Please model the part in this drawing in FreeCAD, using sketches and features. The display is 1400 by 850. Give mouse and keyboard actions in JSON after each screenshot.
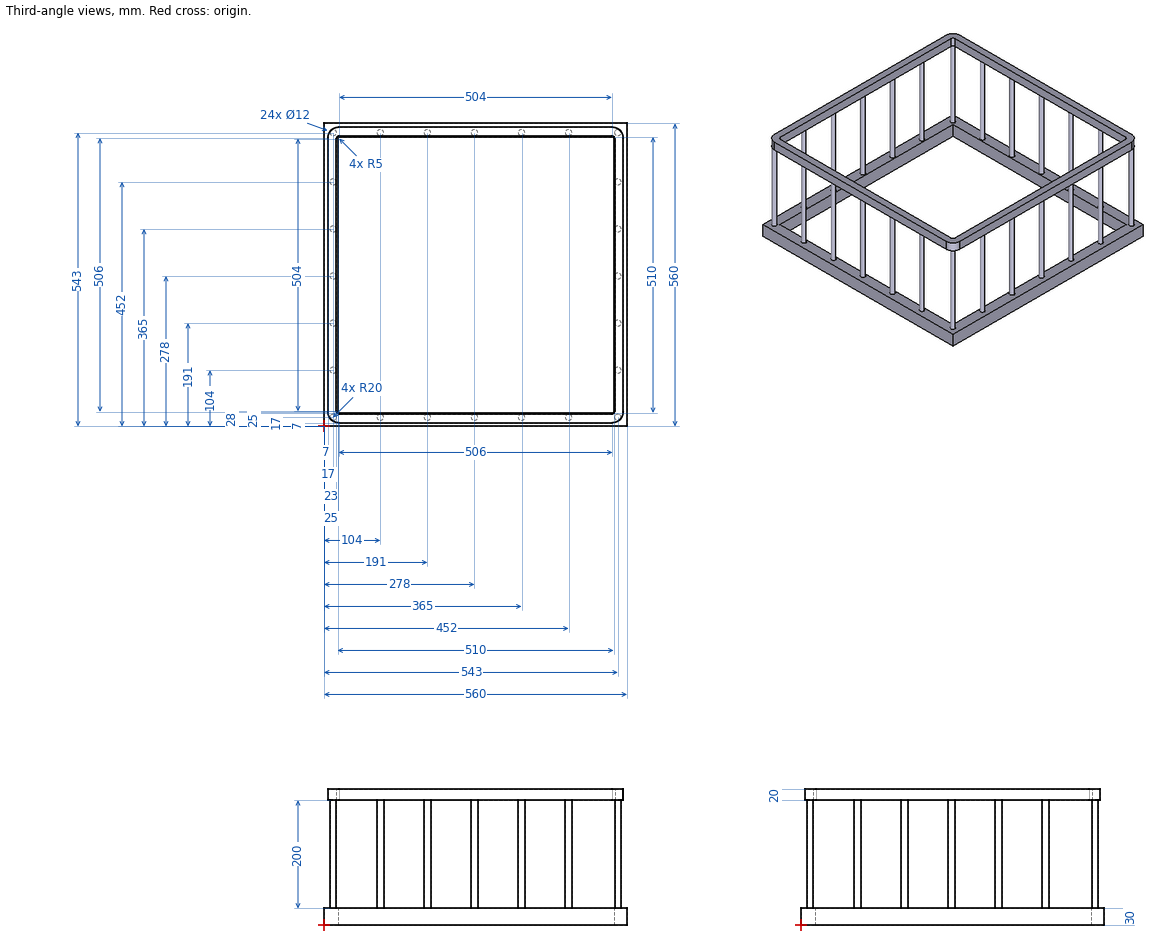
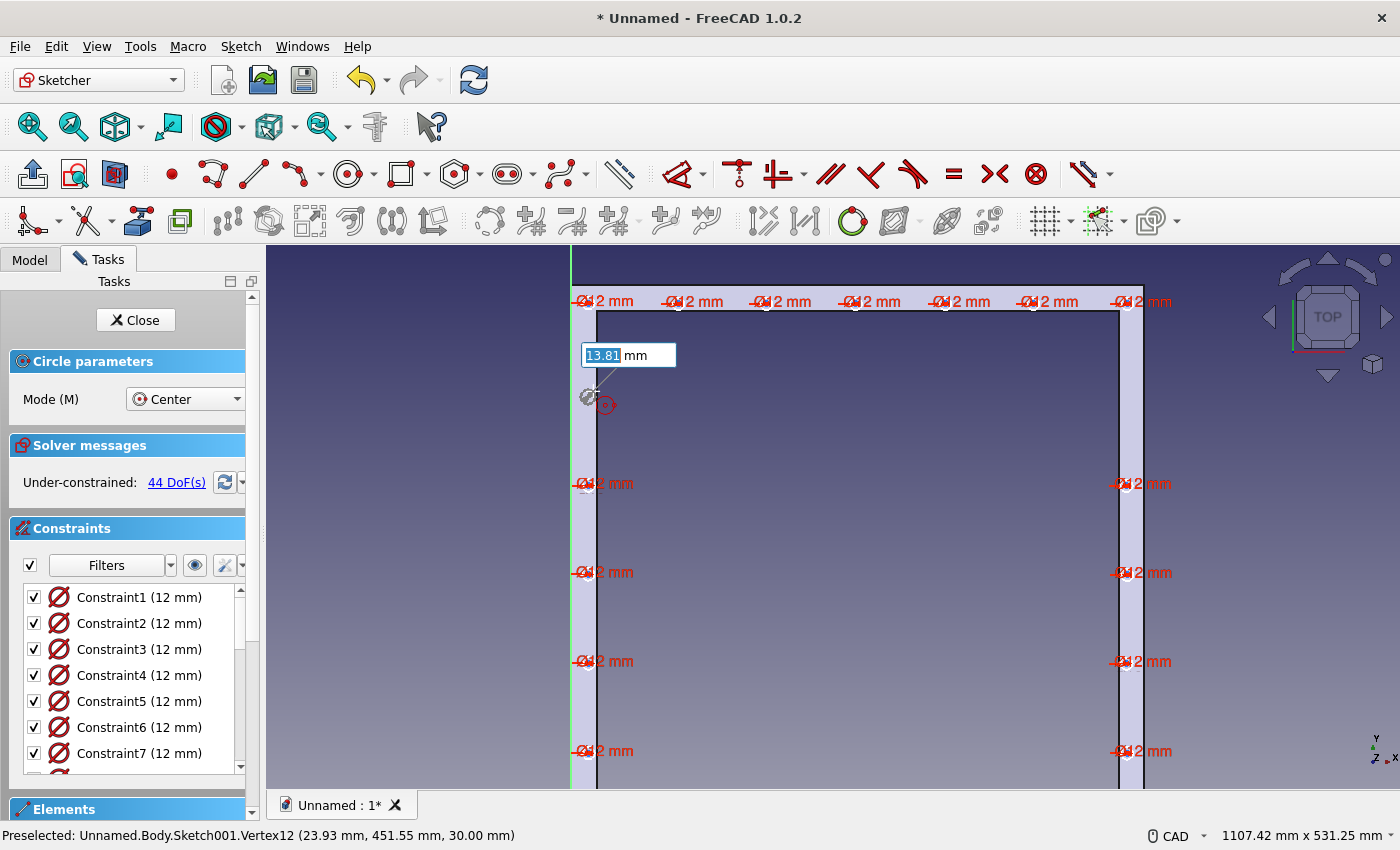
{"action": "type", "text": "12"}
{"action": "key", "text": "Return"}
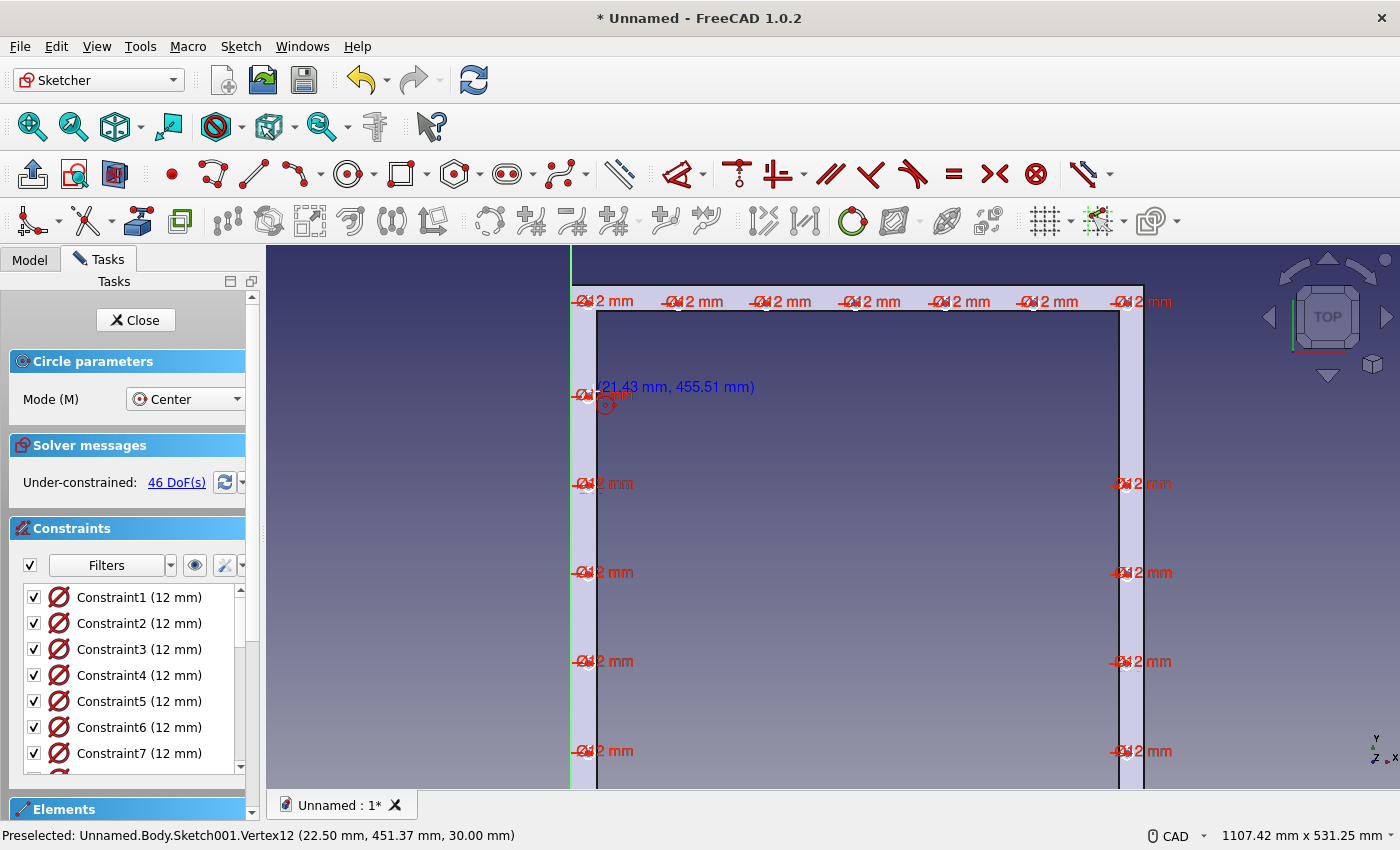
{"action": "scroll", "coordinate": [1127, 396], "scroll_direction": "up", "scroll_amount": 7}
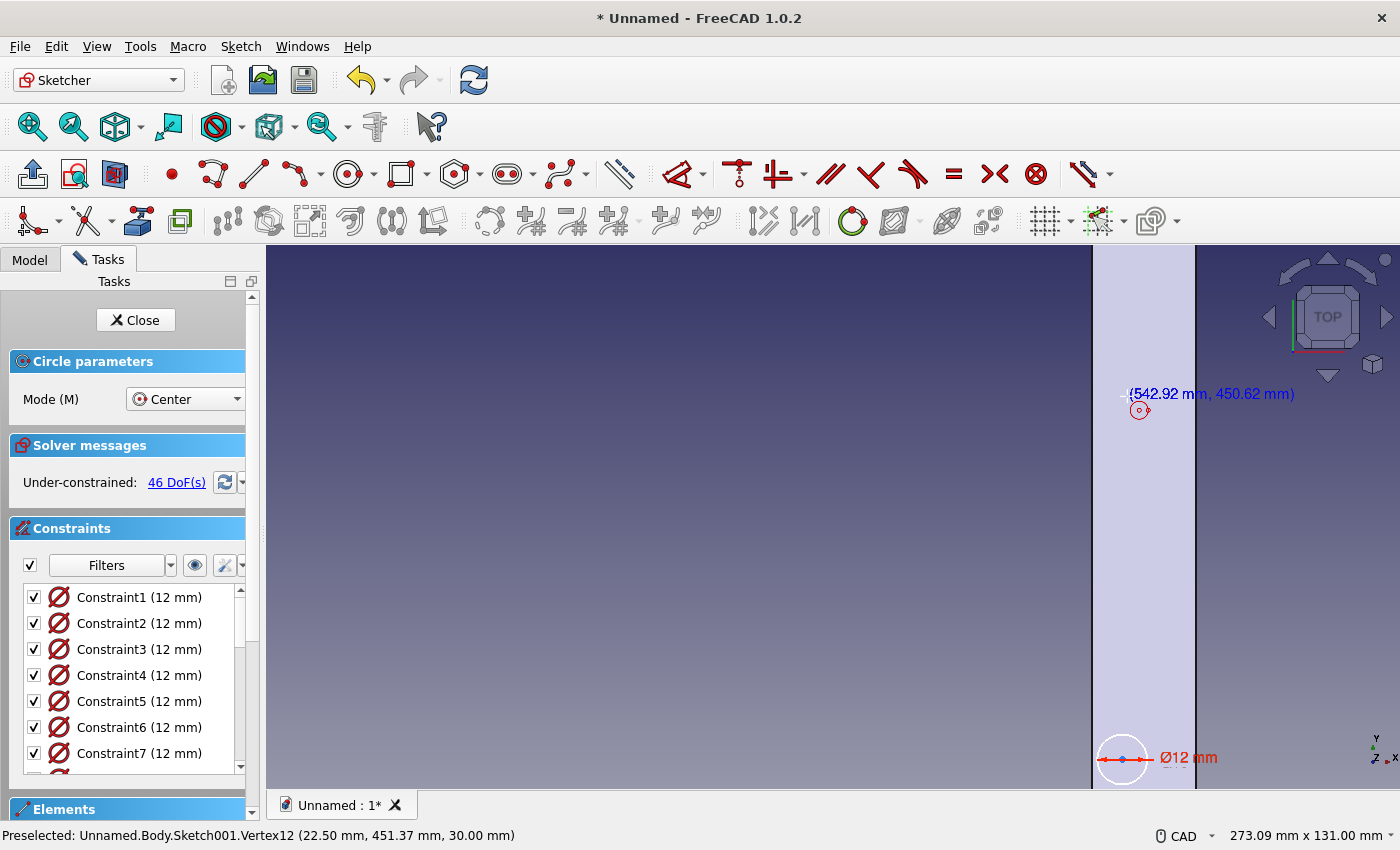
{"action": "scroll", "coordinate": [914, 395], "scroll_direction": "down", "scroll_amount": 9}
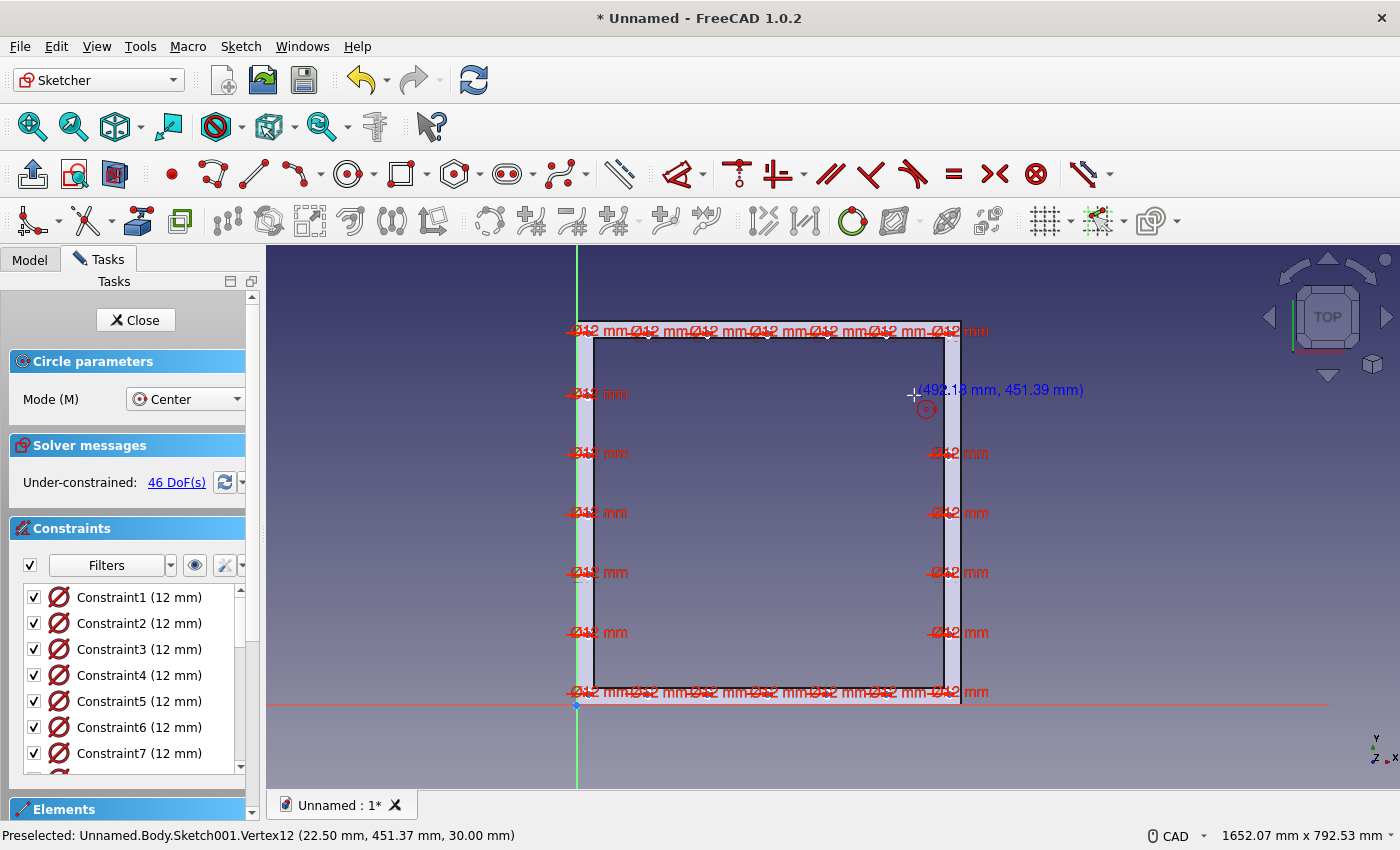
{"action": "left_click", "coordinate": [949, 395]}
{"action": "mouse_move", "coordinate": [952, 392]}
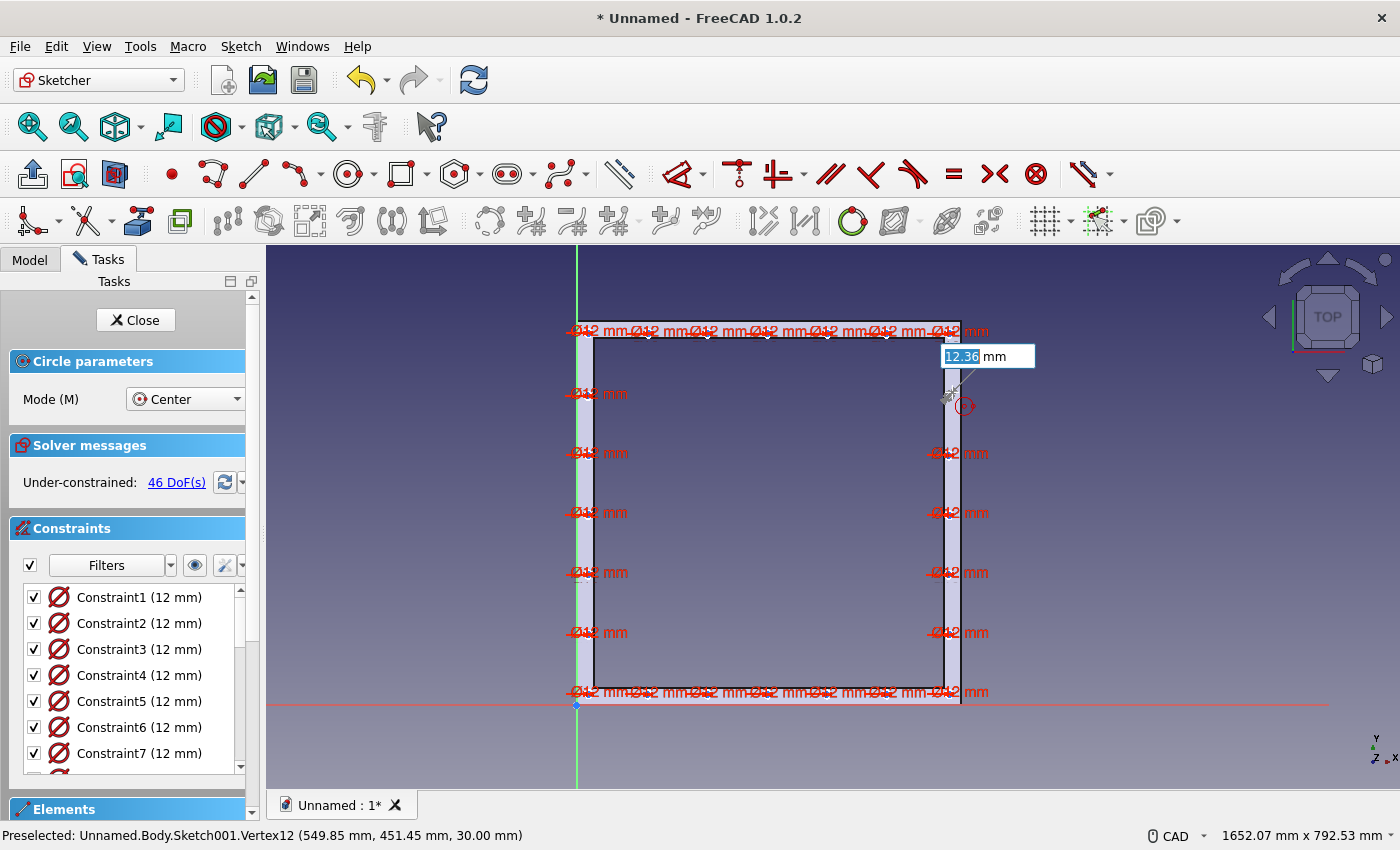
{"action": "type", "text": "12"}
{"action": "key", "text": "Return"}
{"action": "key", "text": "Escape"}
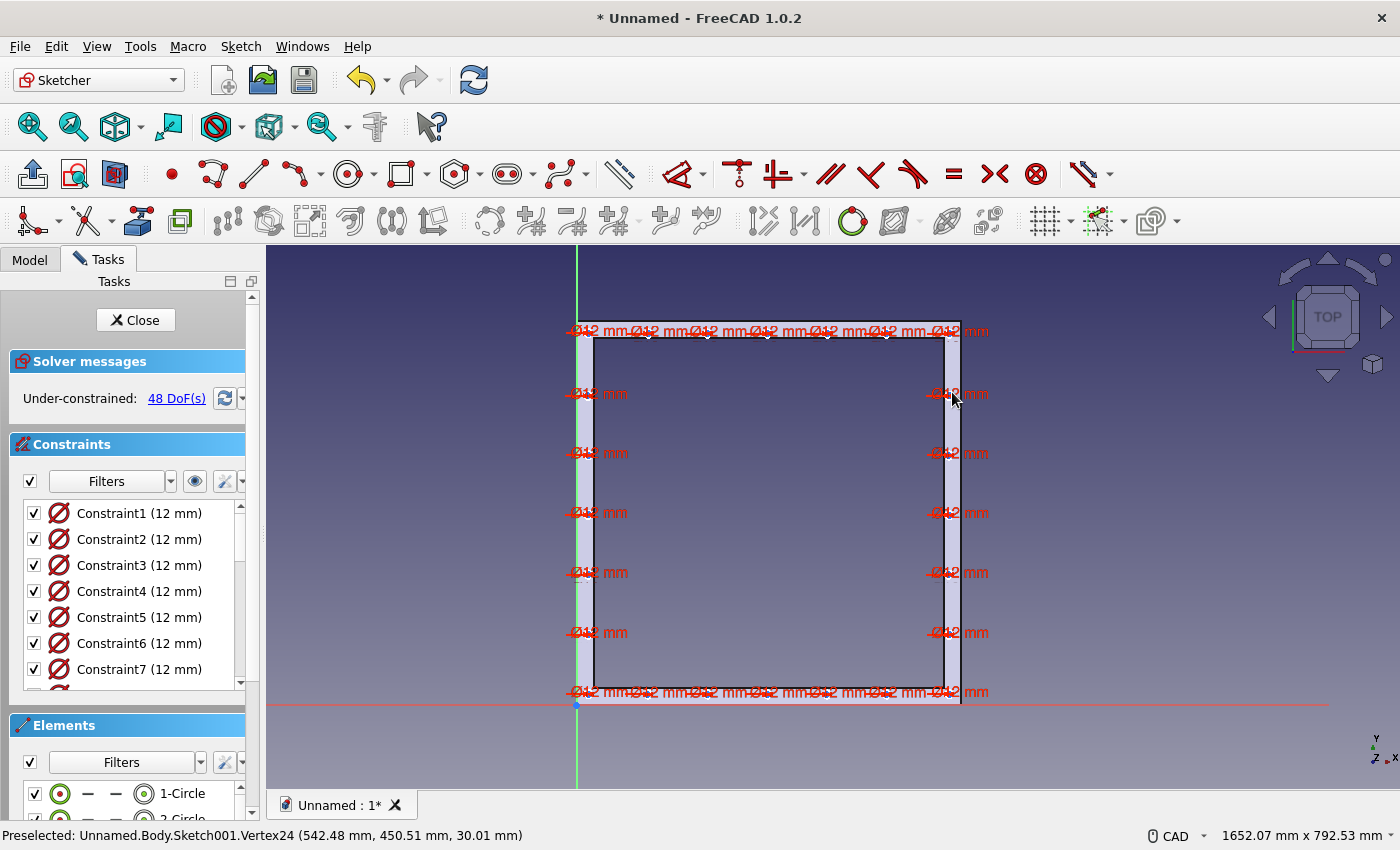
{"action": "left_click", "coordinate": [588, 333]}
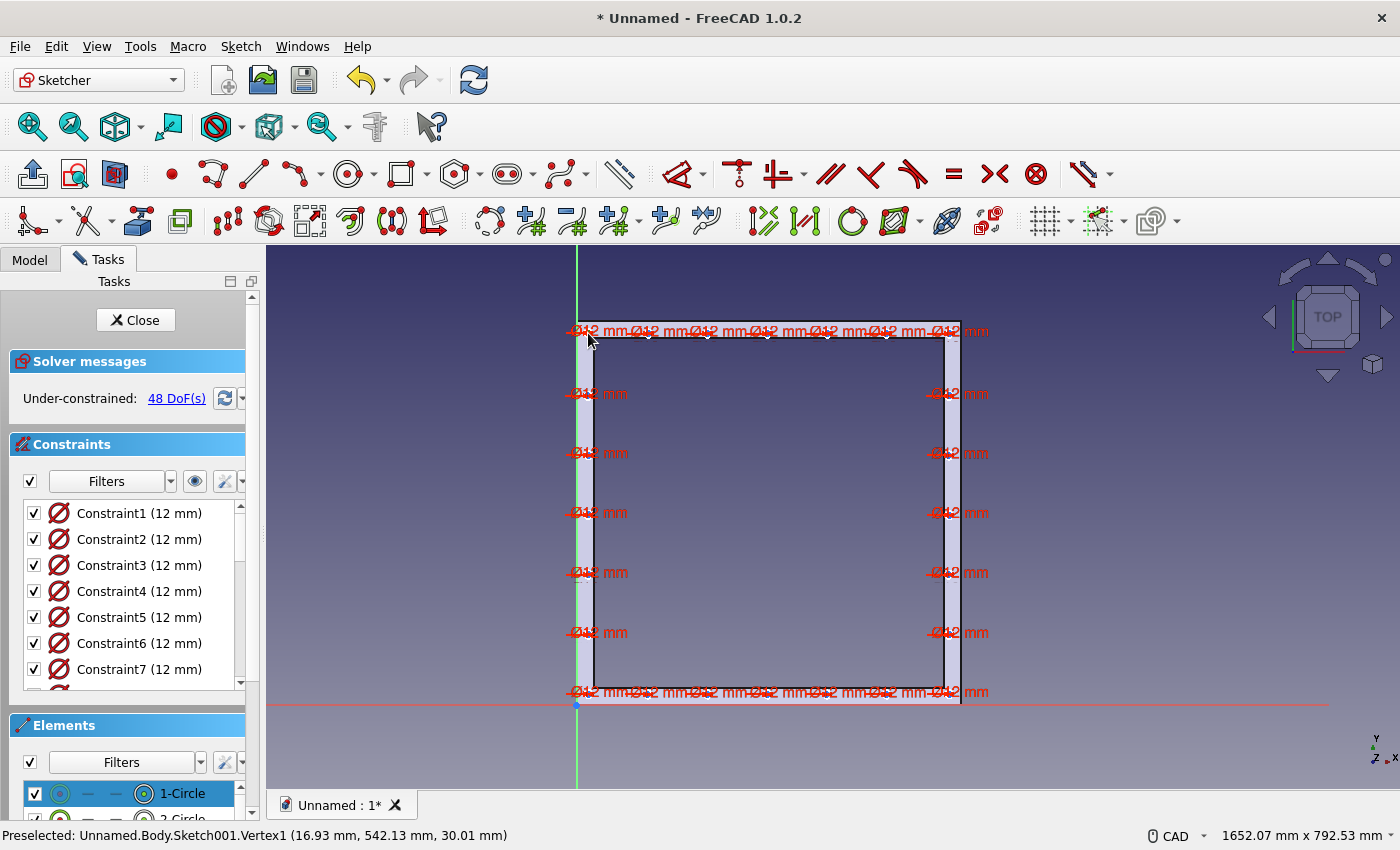
{"action": "left_click", "coordinate": [589, 694]}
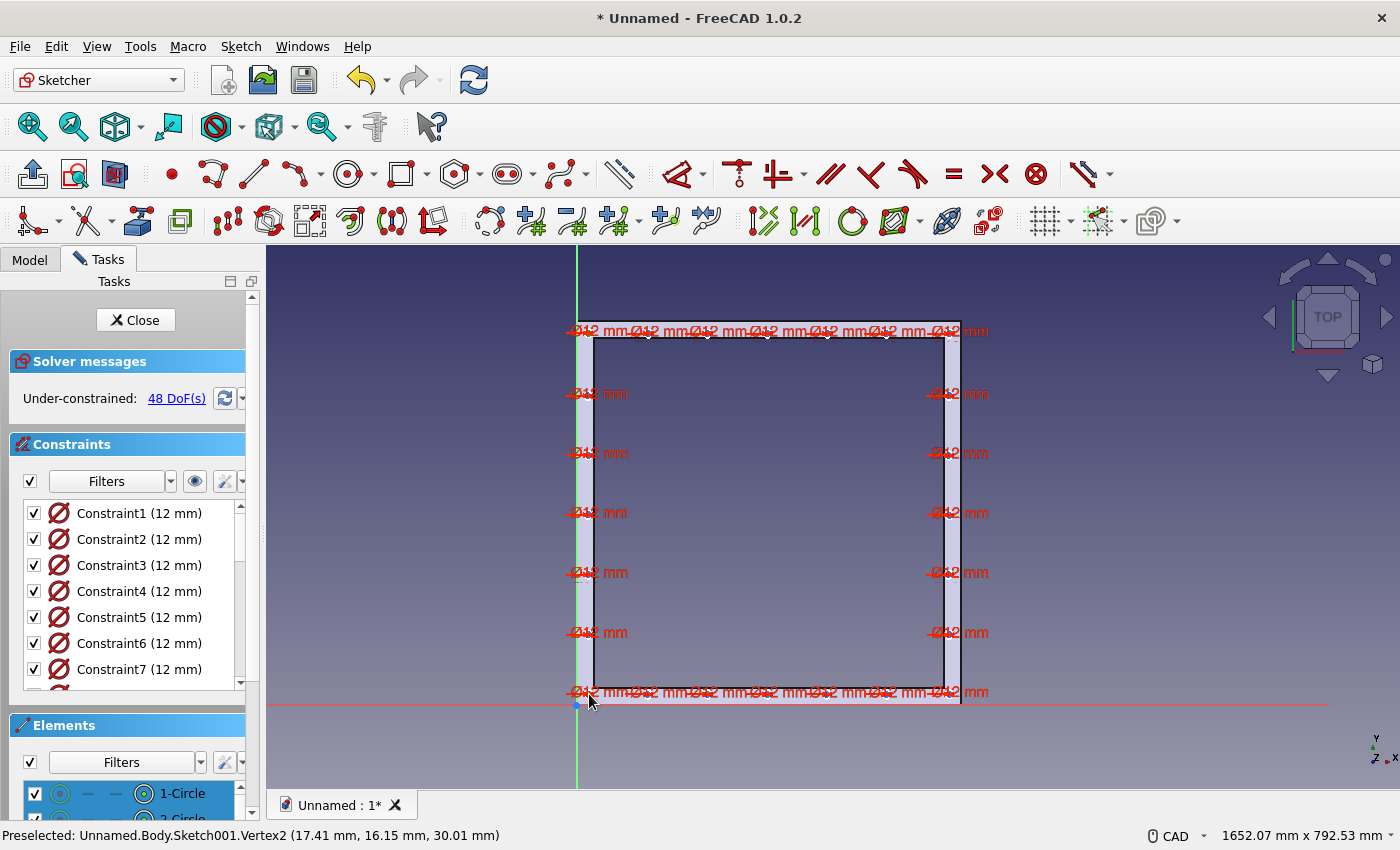
{"action": "key", "text": "v"}